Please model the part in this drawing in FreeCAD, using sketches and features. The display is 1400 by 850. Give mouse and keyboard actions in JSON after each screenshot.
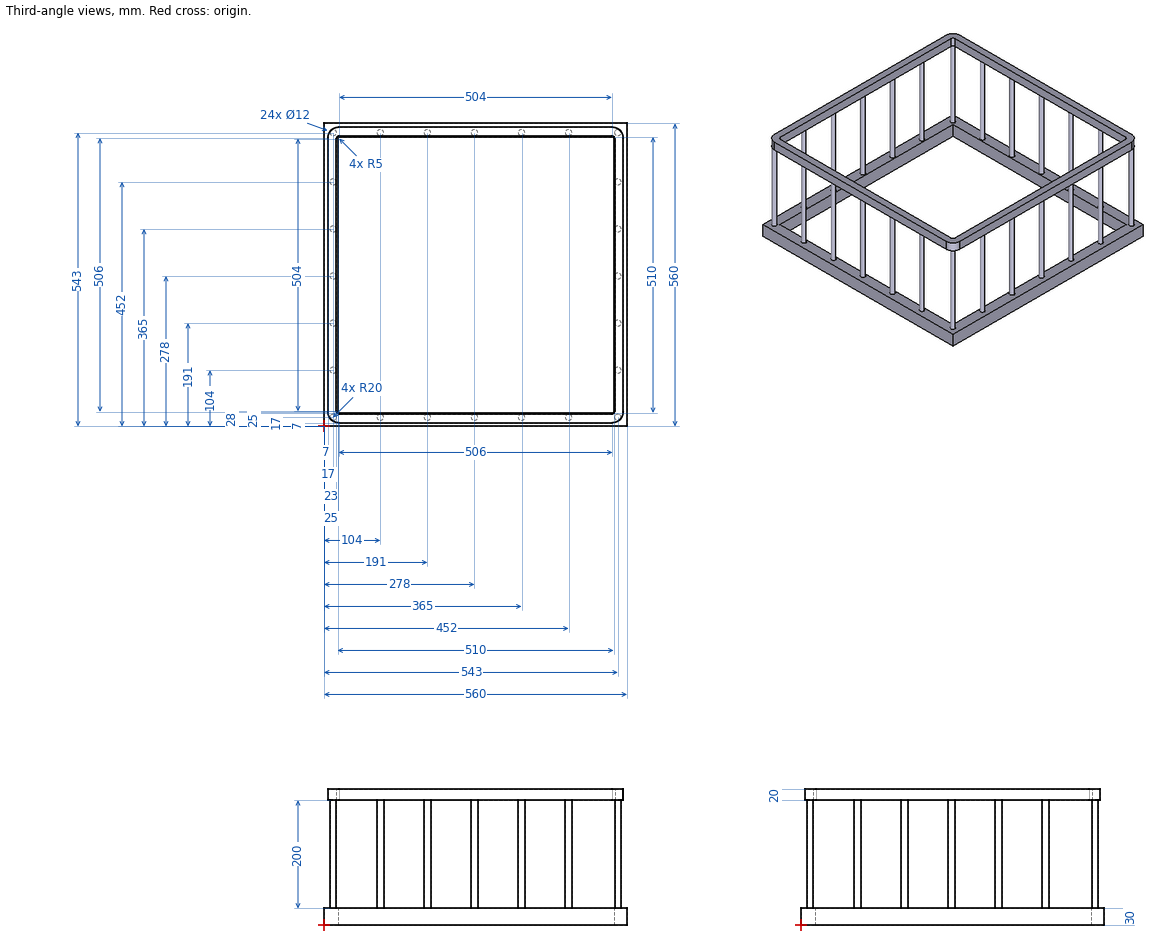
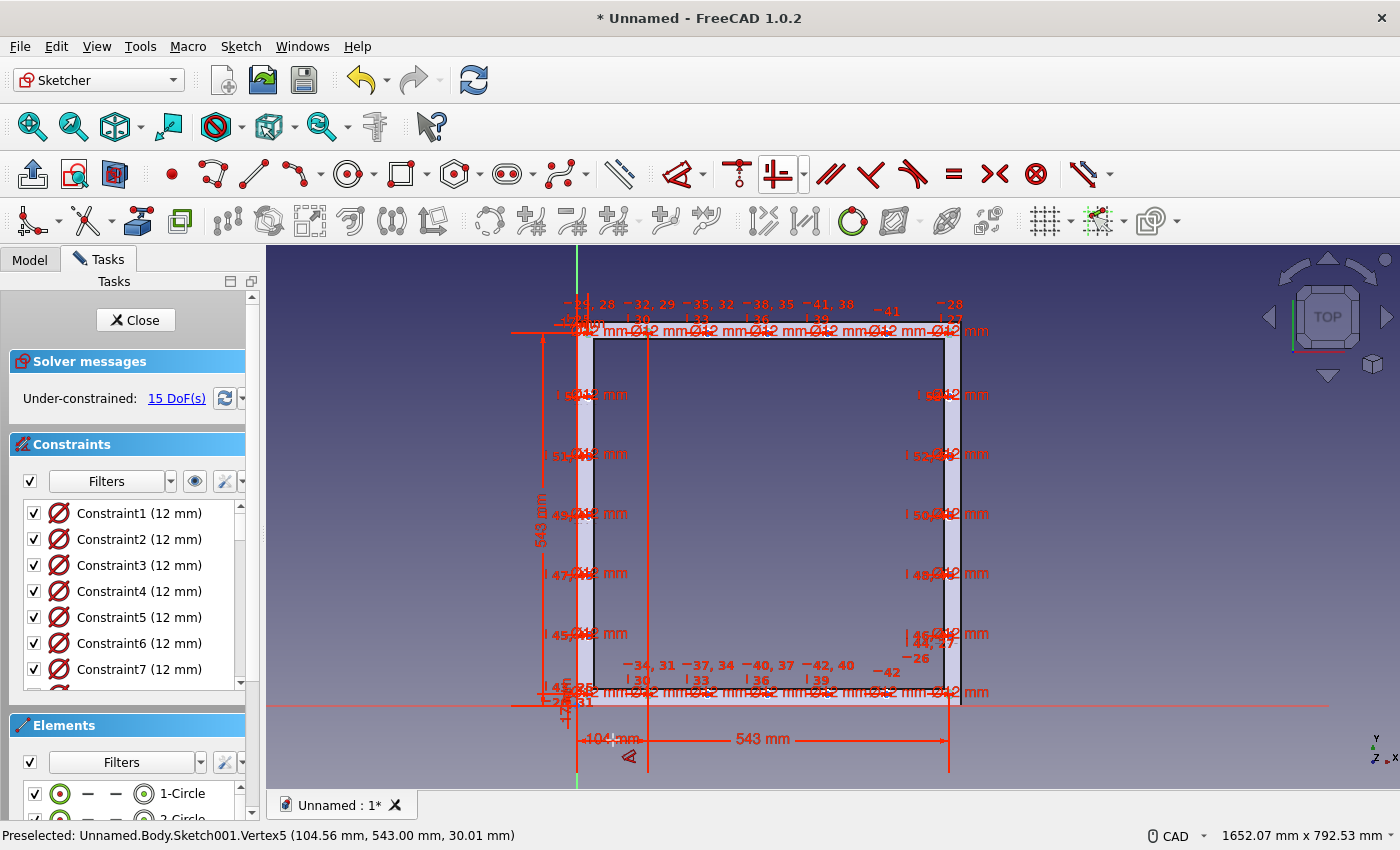
{"action": "left_click", "coordinate": [707, 333]}
{"action": "left_click", "coordinate": [688, 740]}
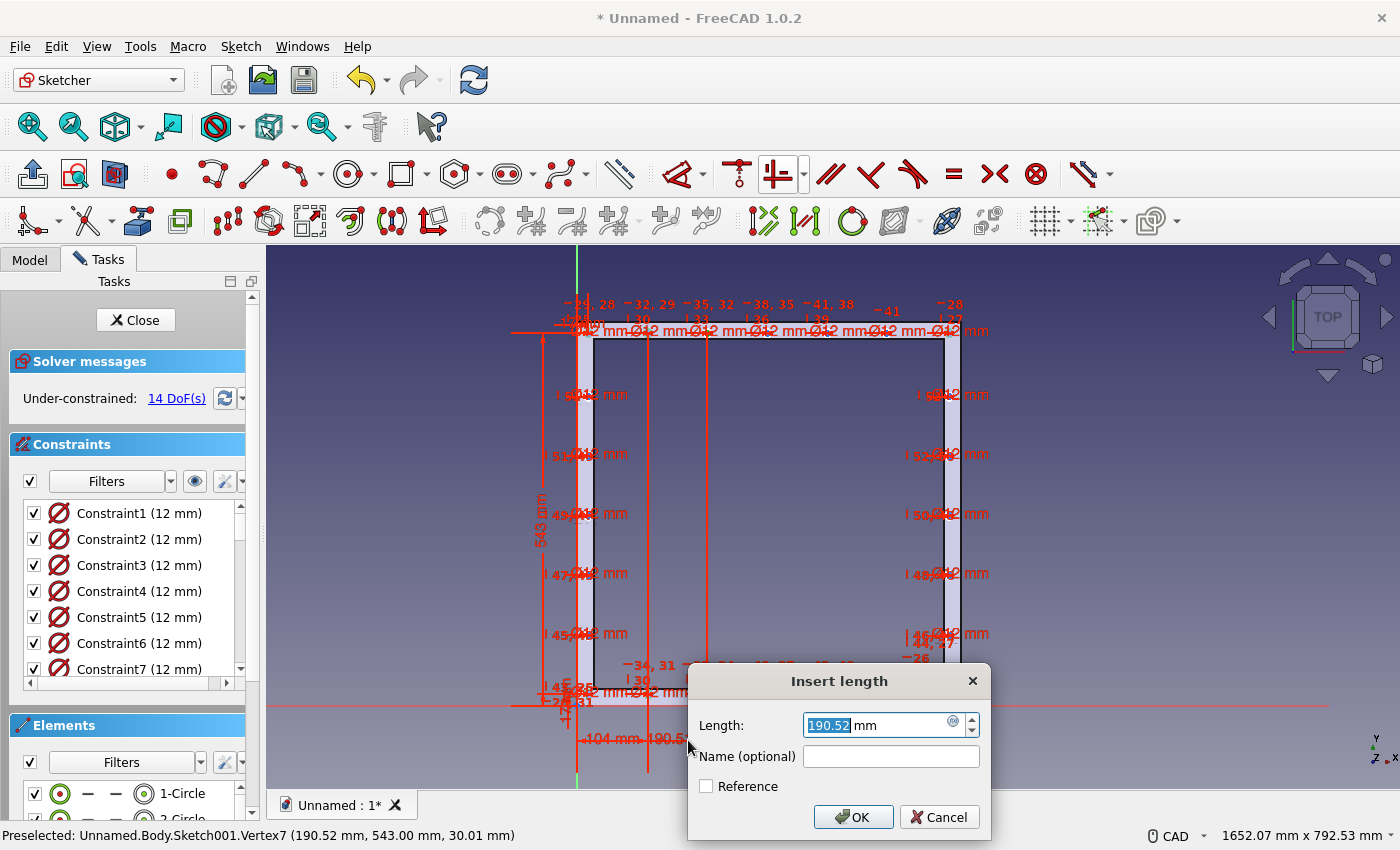
{"action": "type", "text": "191"}
{"action": "key", "text": "Return"}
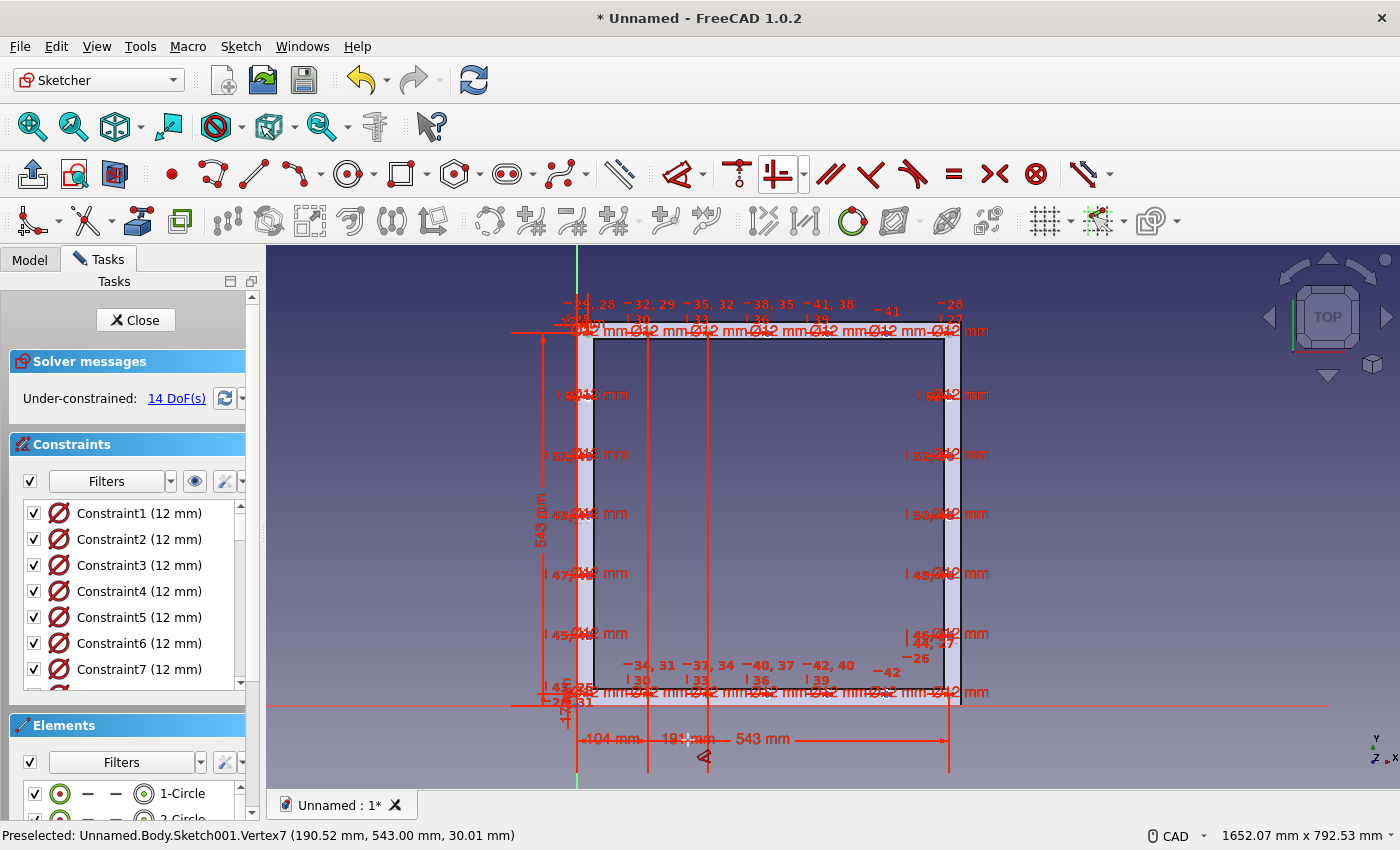
{"action": "left_click", "coordinate": [767, 333]}
{"action": "left_click", "coordinate": [672, 299]}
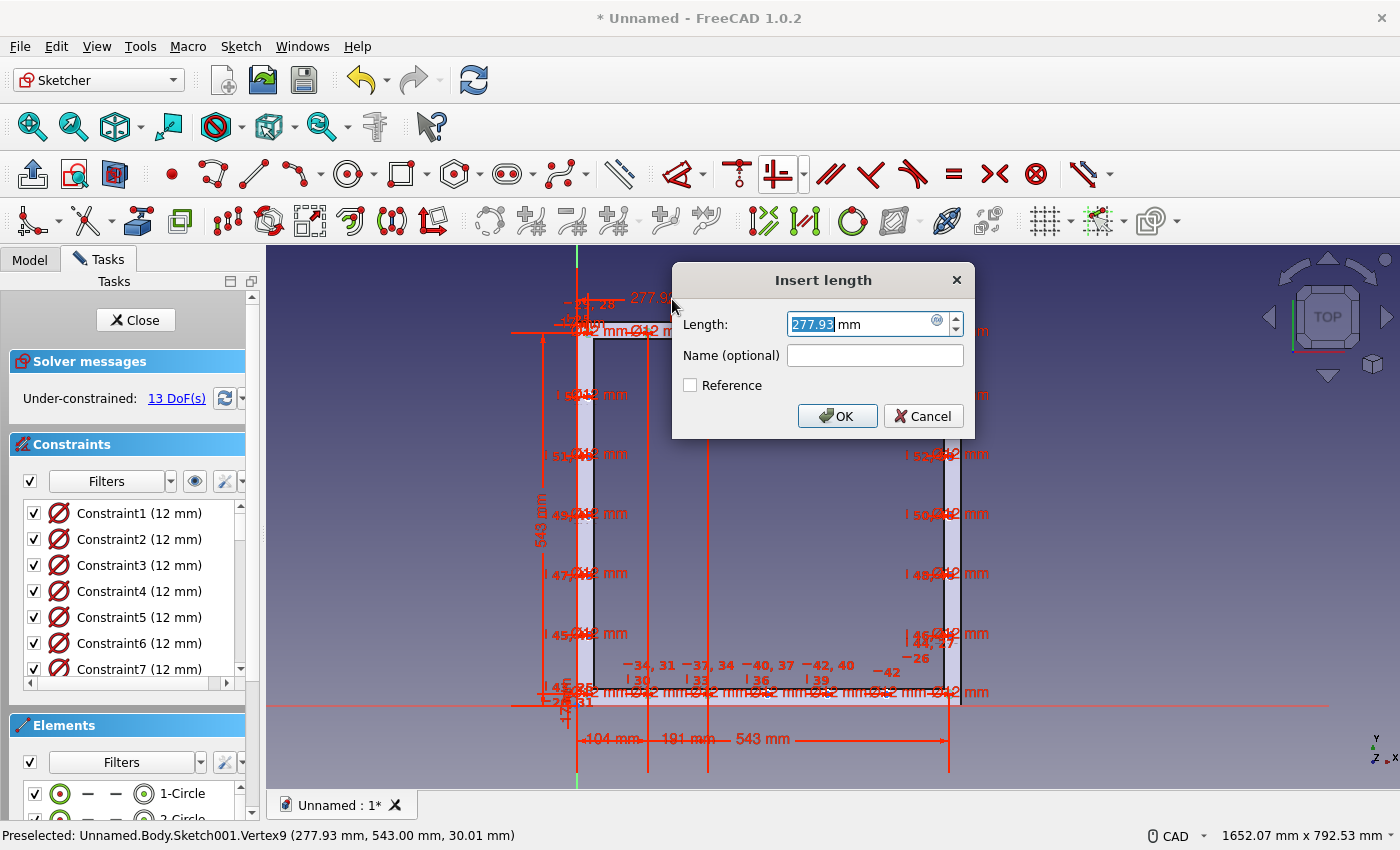
{"action": "type", "text": "278"}
{"action": "key", "text": "Return"}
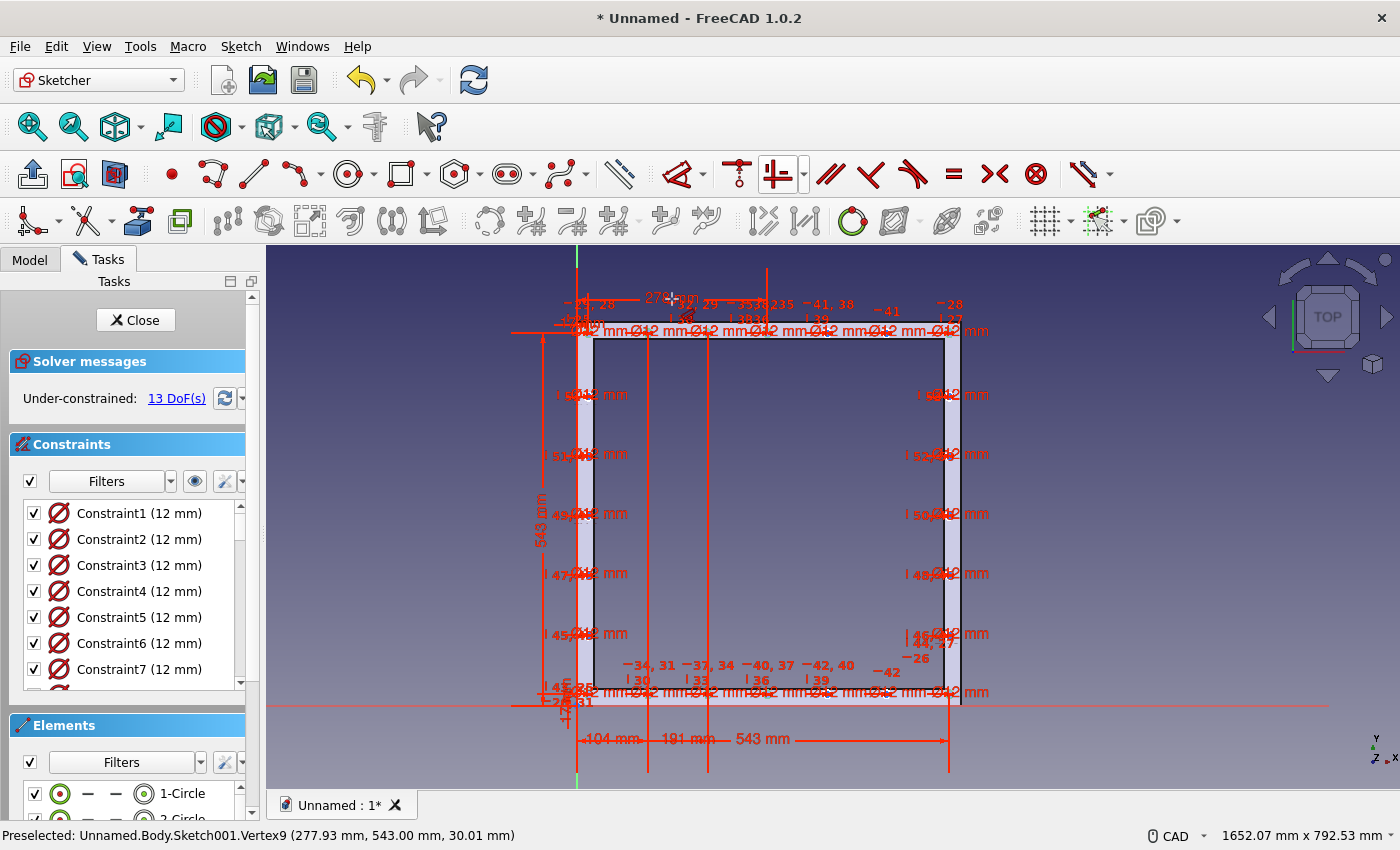
{"action": "left_click", "coordinate": [827, 333]}
{"action": "left_click", "coordinate": [760, 299]}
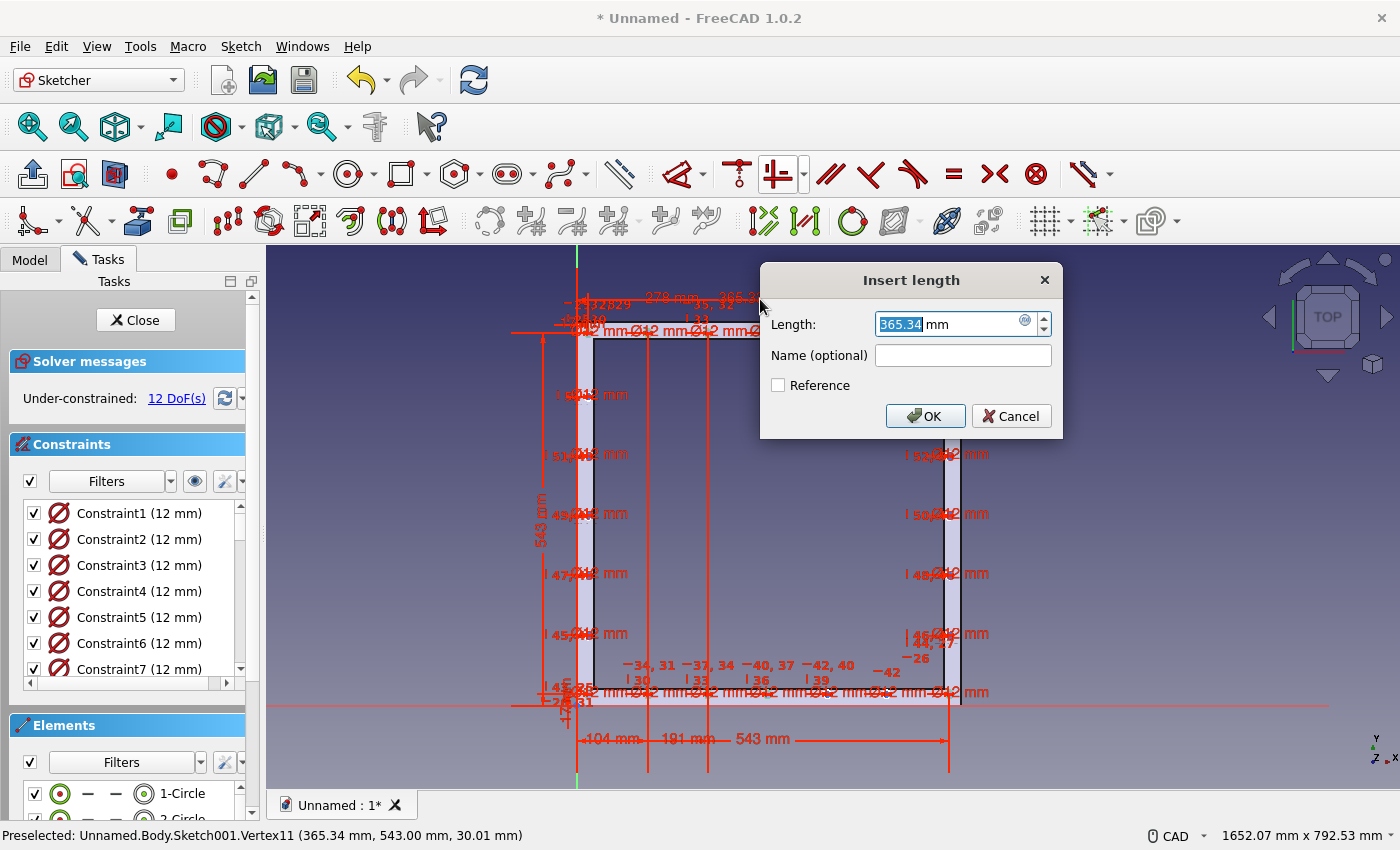
{"action": "type", "text": "365"}
{"action": "key", "text": "Return"}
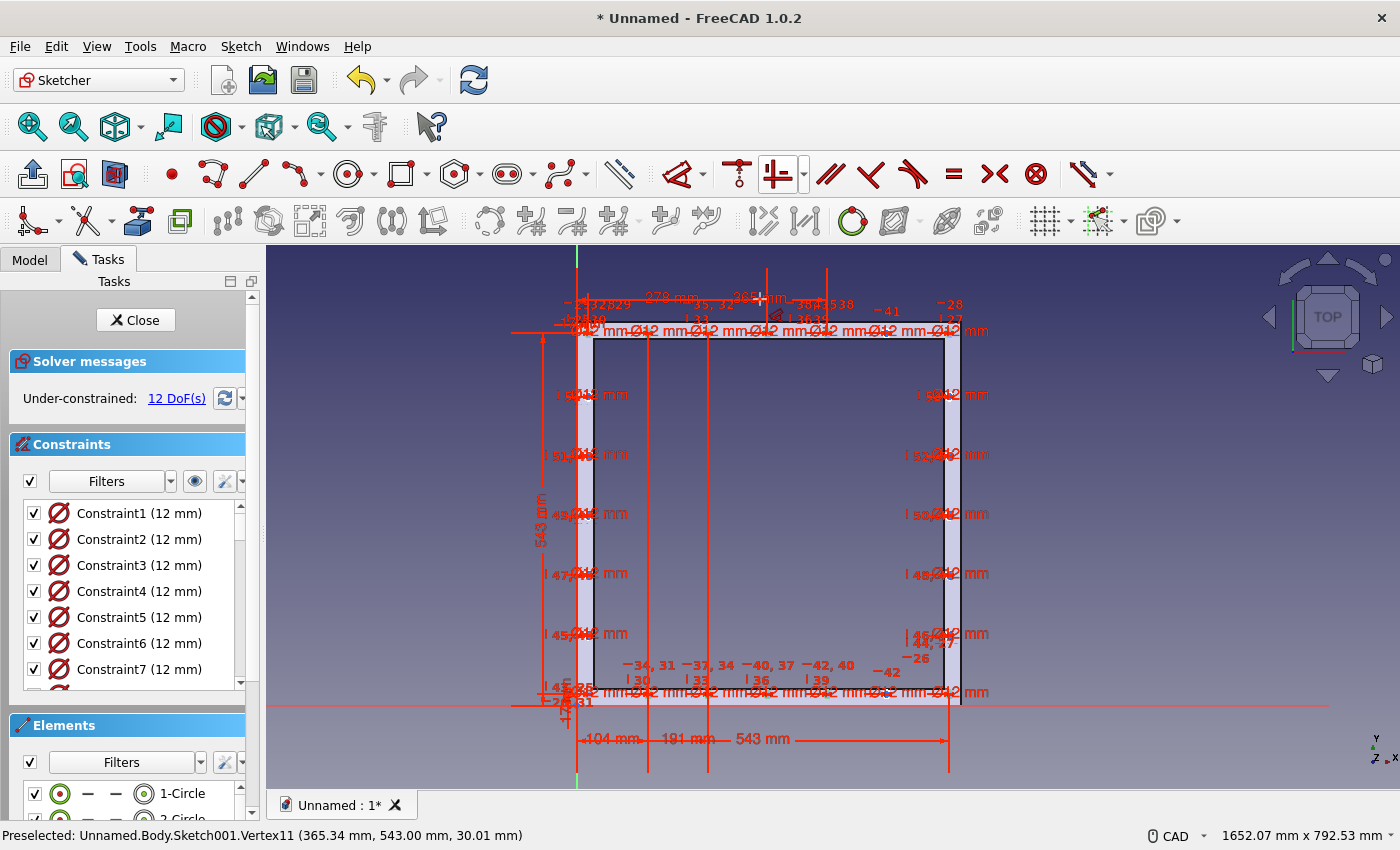
{"action": "left_click", "coordinate": [886, 333]}
{"action": "left_click", "coordinate": [840, 740]}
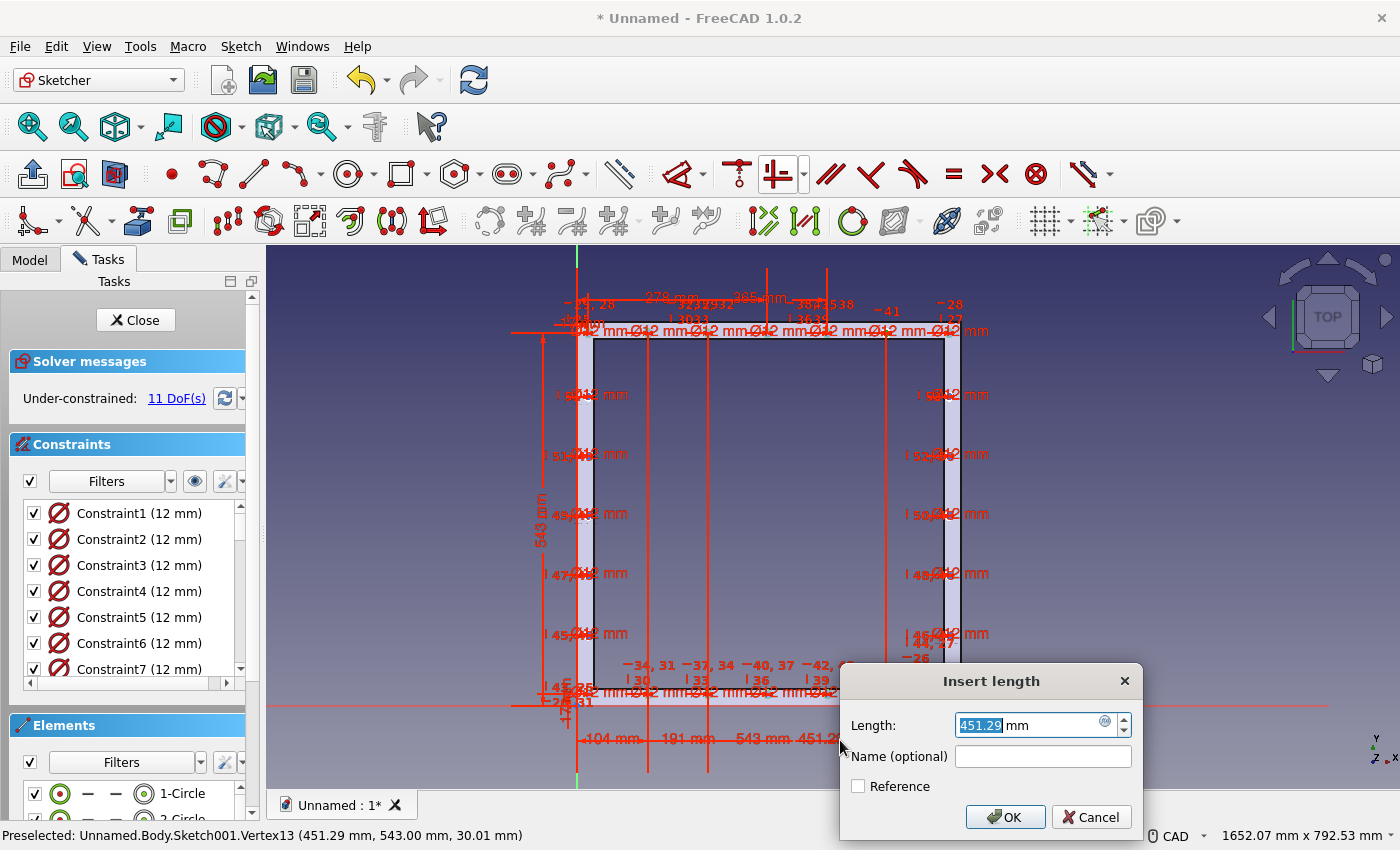
{"action": "type", "text": "452"}
{"action": "key", "text": "Return"}